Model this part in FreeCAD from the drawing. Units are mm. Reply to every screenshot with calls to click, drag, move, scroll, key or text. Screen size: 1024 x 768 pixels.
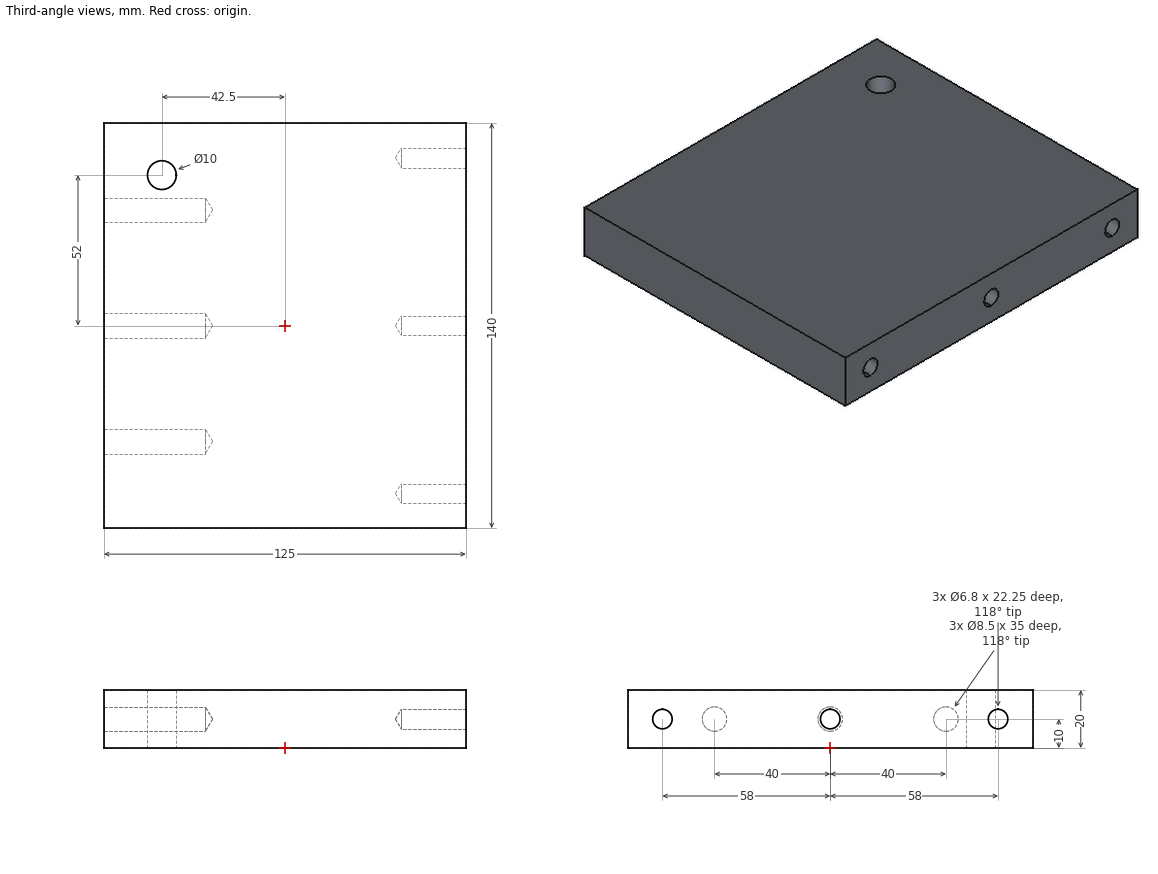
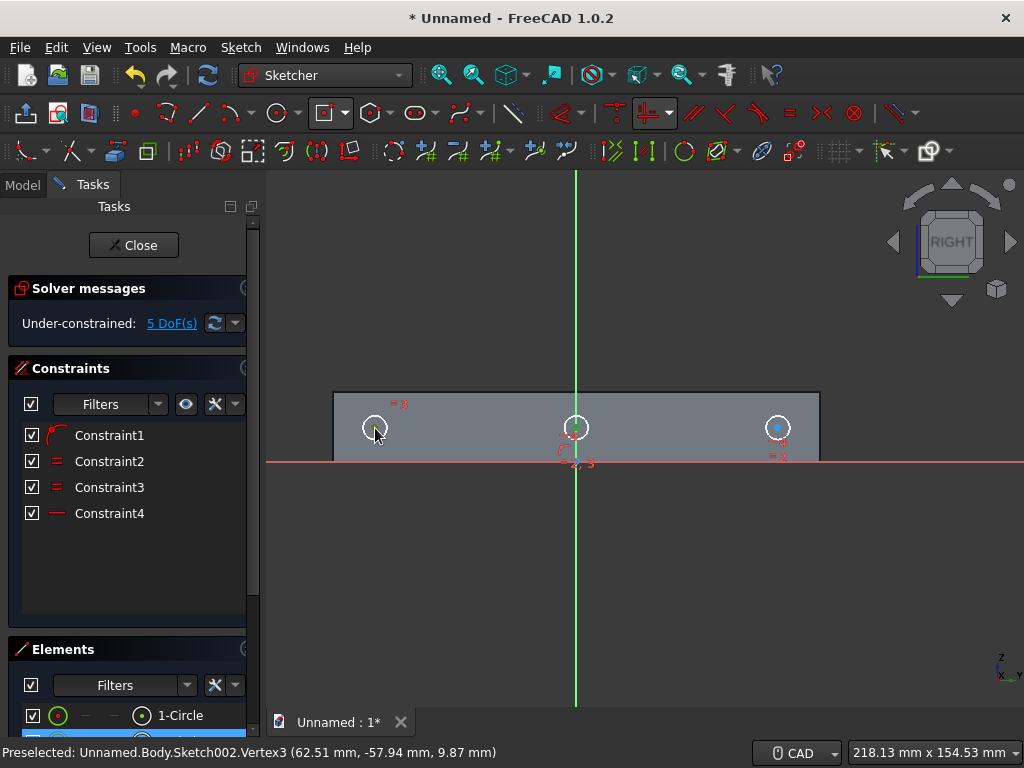
key(h)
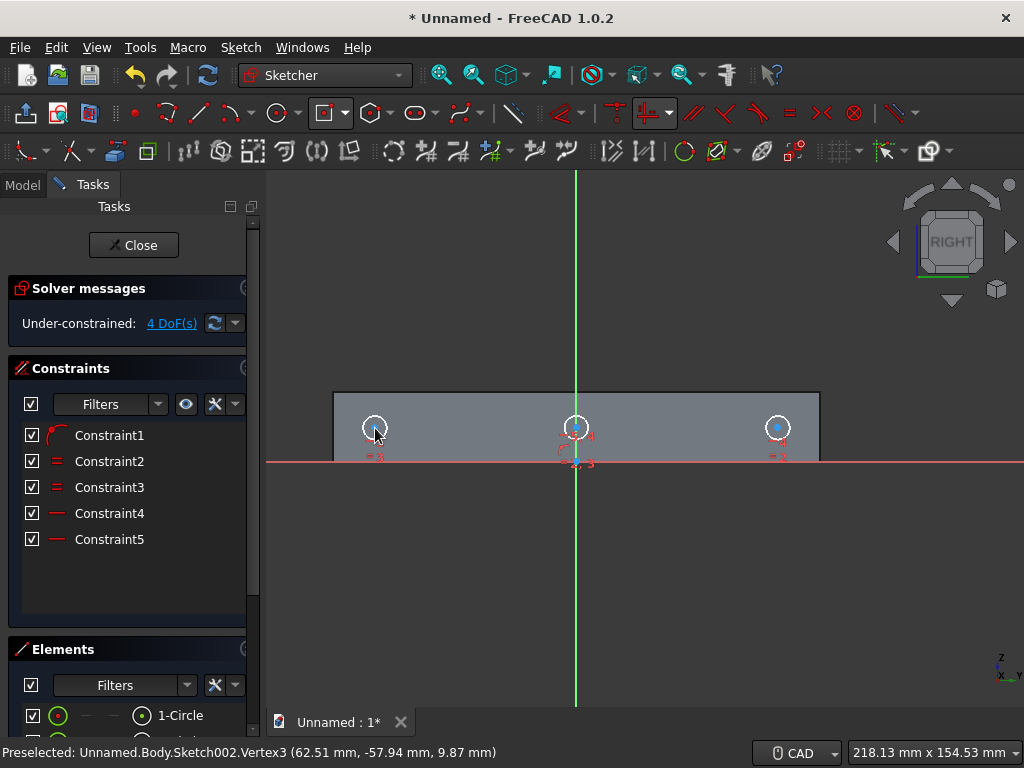
click(560, 114)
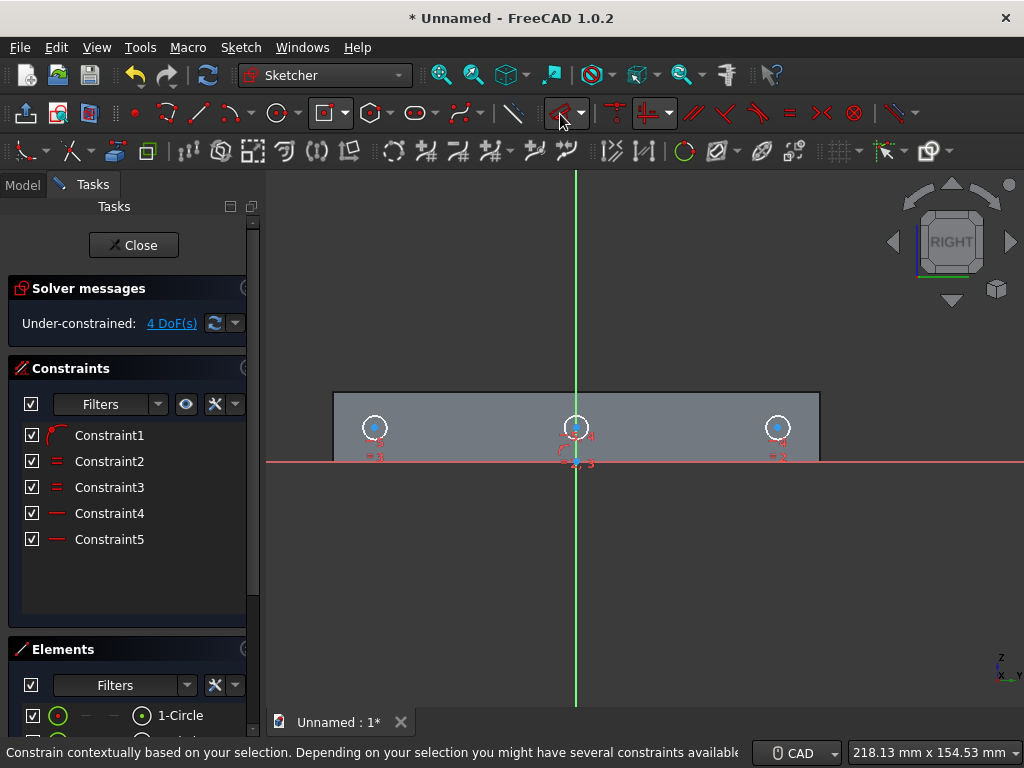
scroll(786, 419, up, 3)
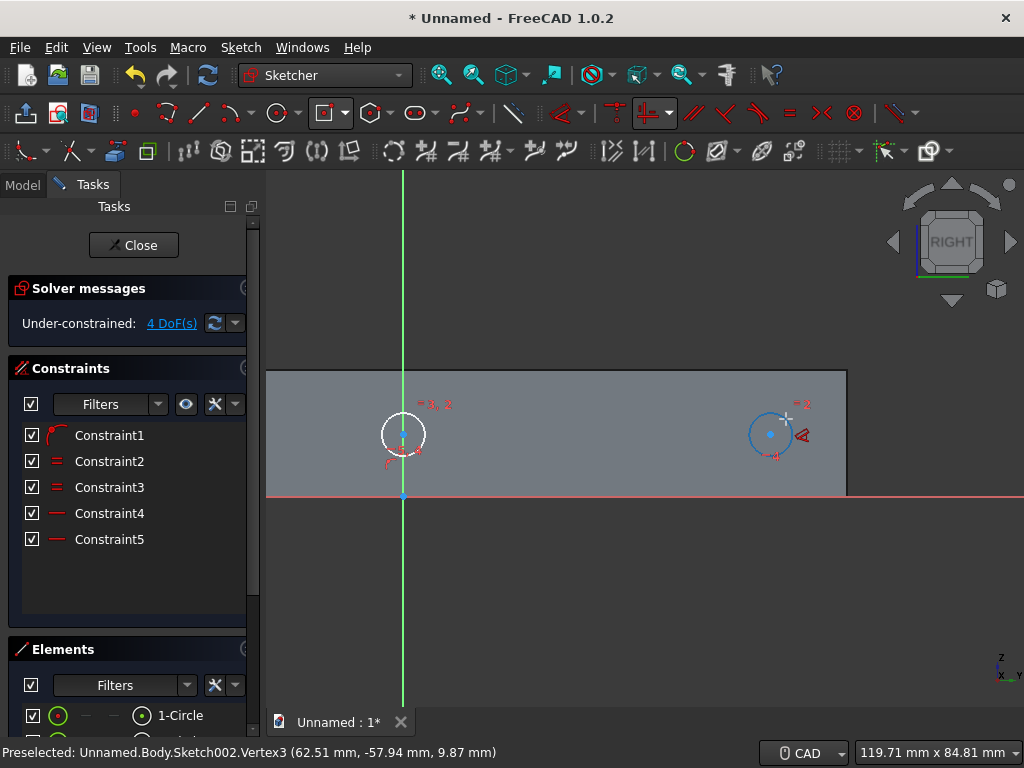
click(786, 419)
click(808, 396)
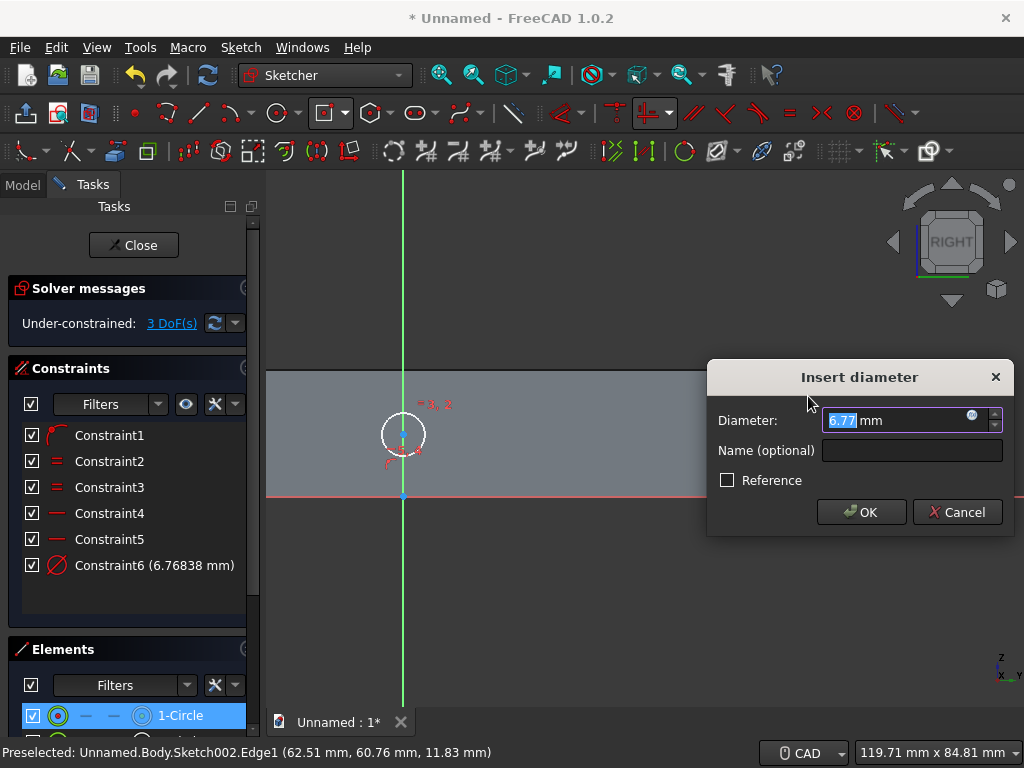
text(6.8)
key(Return)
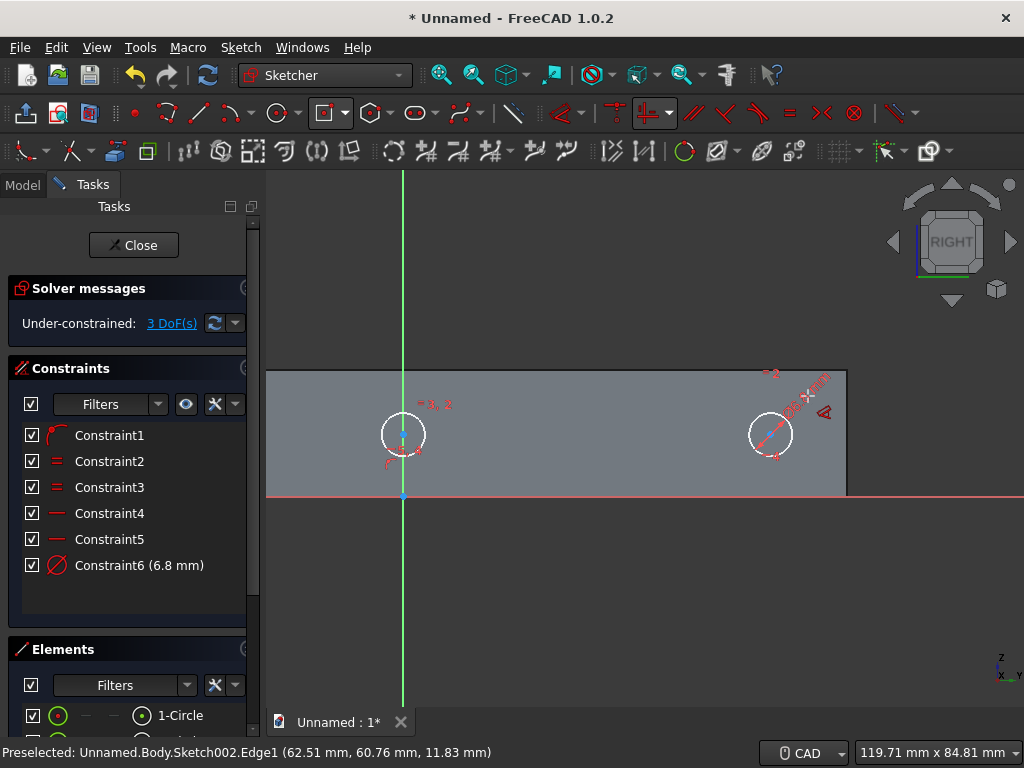
click(771, 435)
click(587, 531)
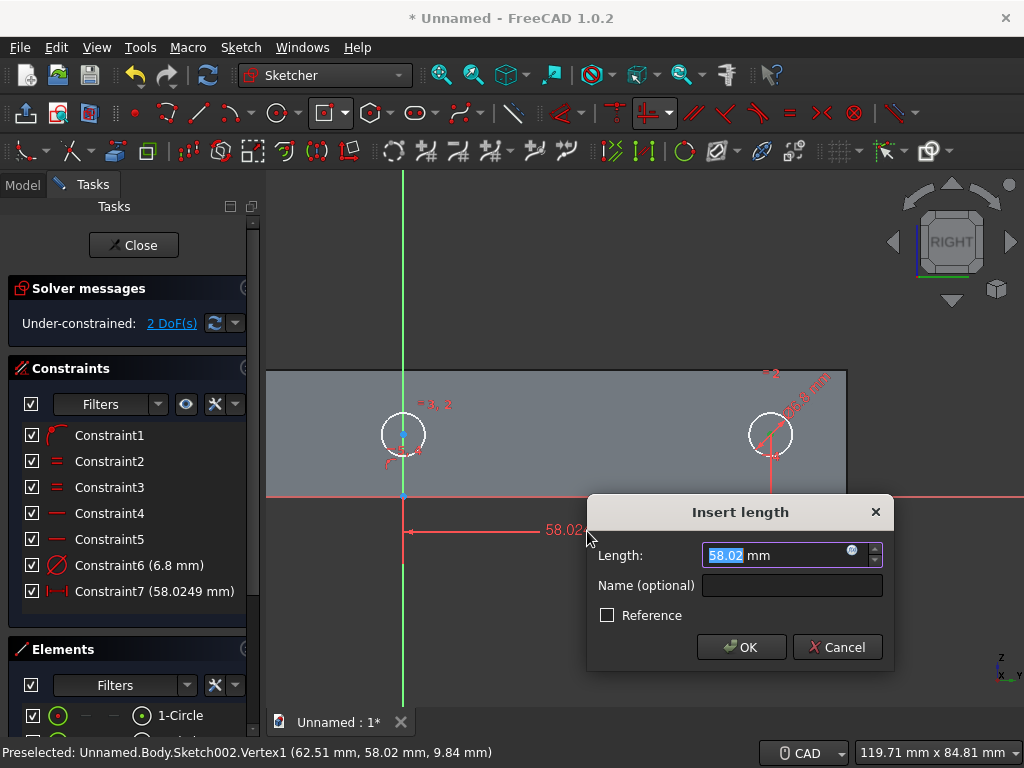
text(58)
key(Return)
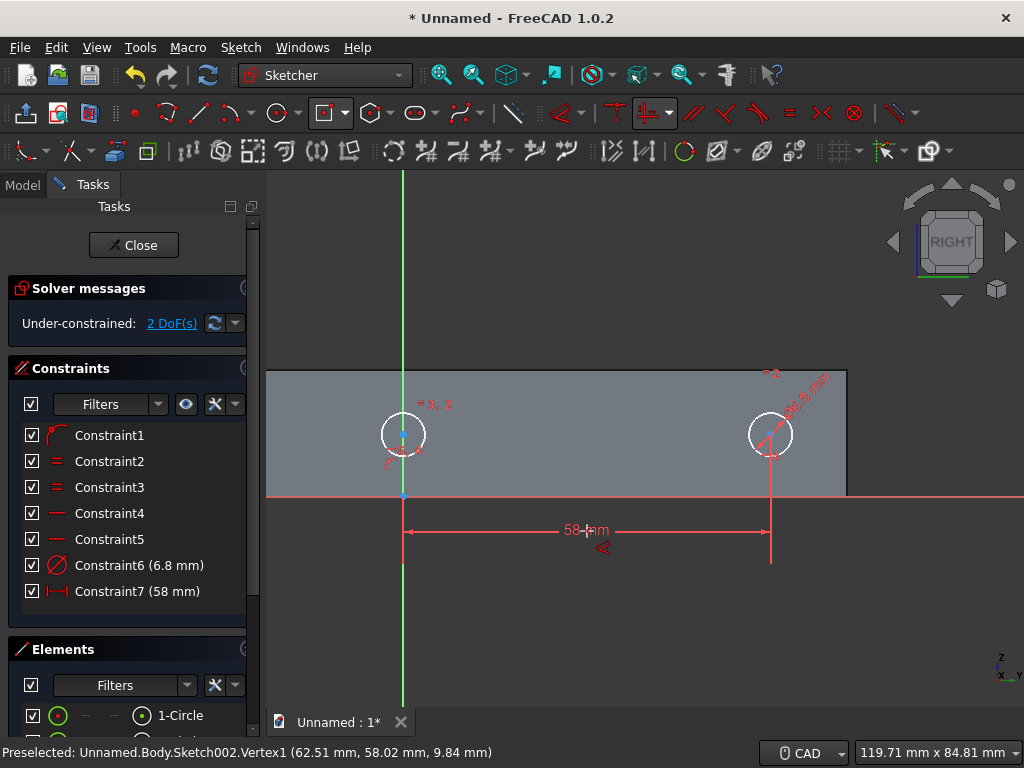
click(771, 435)
click(805, 466)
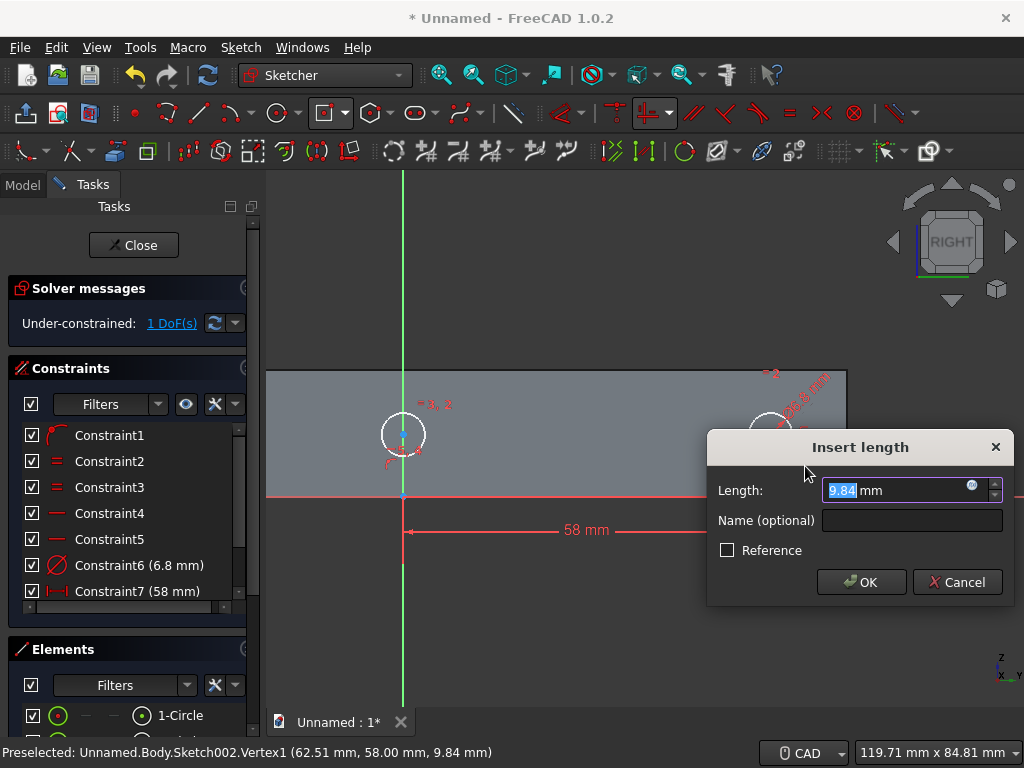
text(10)
key(Return)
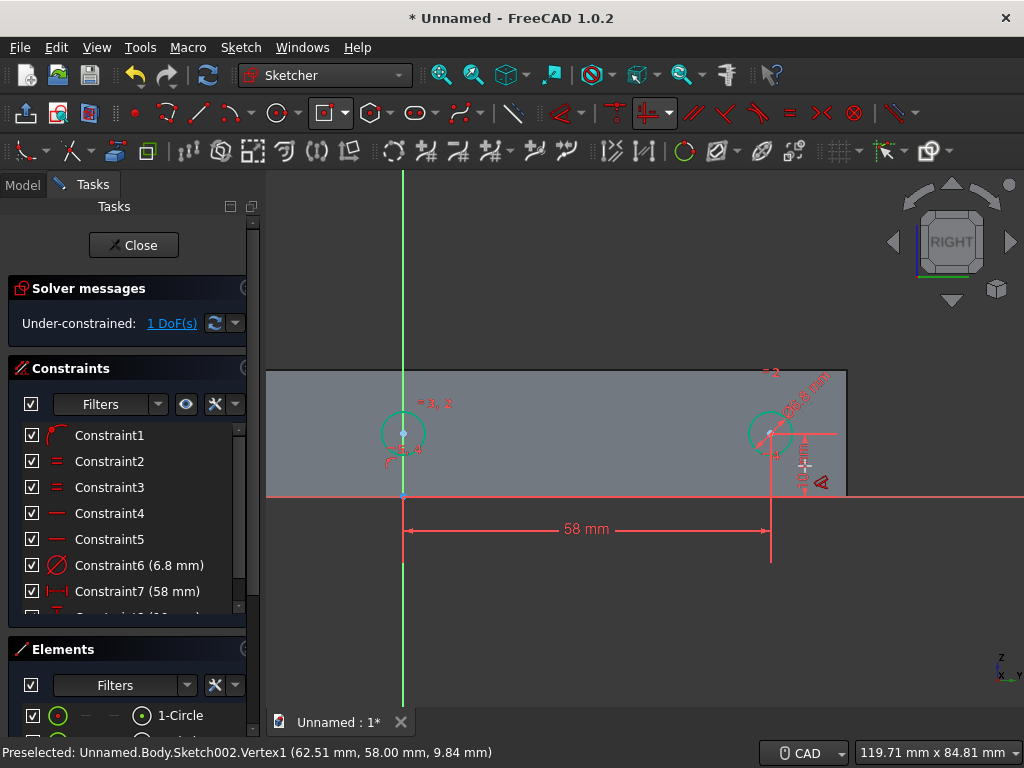
scroll(787, 419, down, 3)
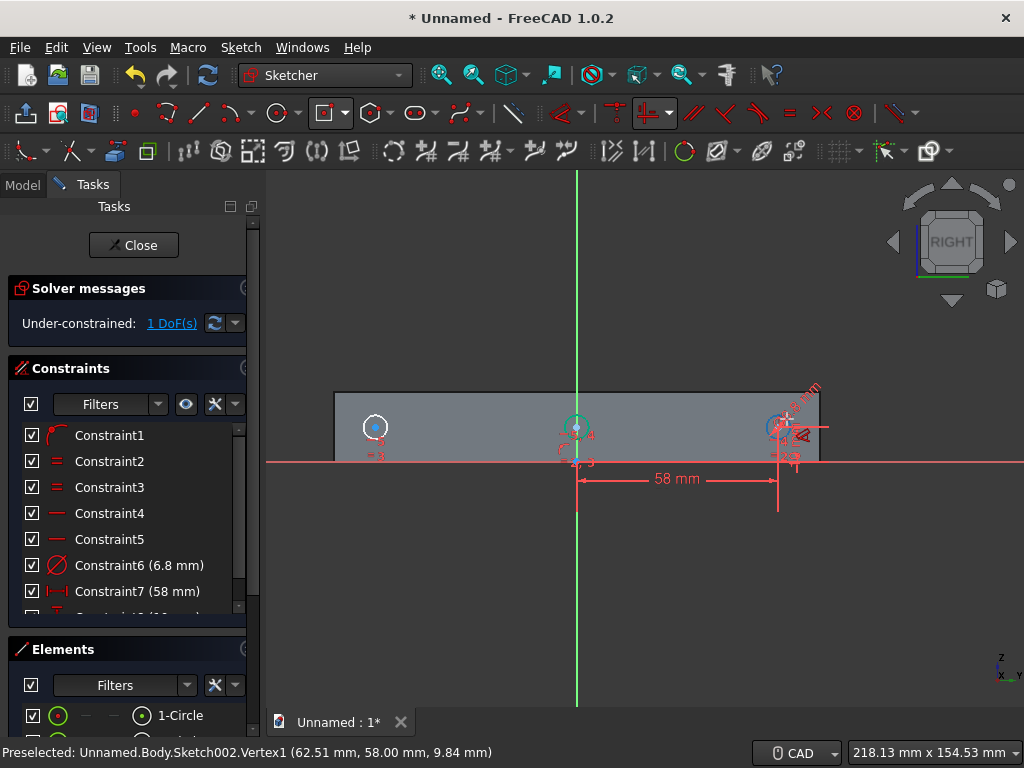
click(375, 427)
click(476, 496)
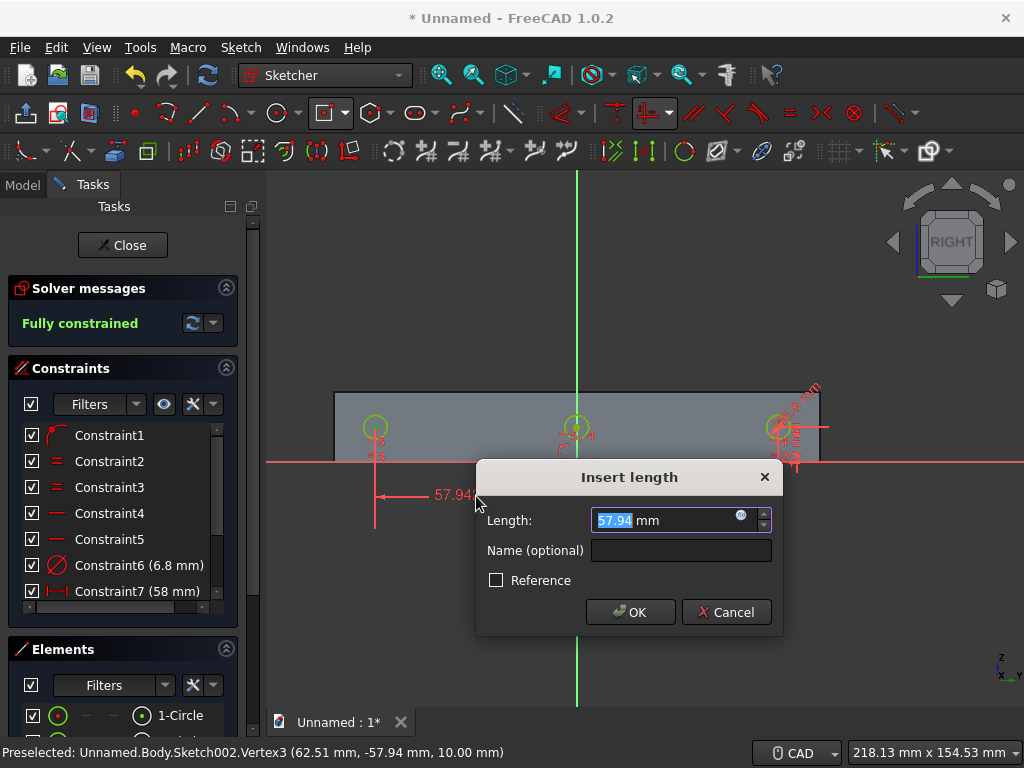
text(58)
key(Return)
key(Escape)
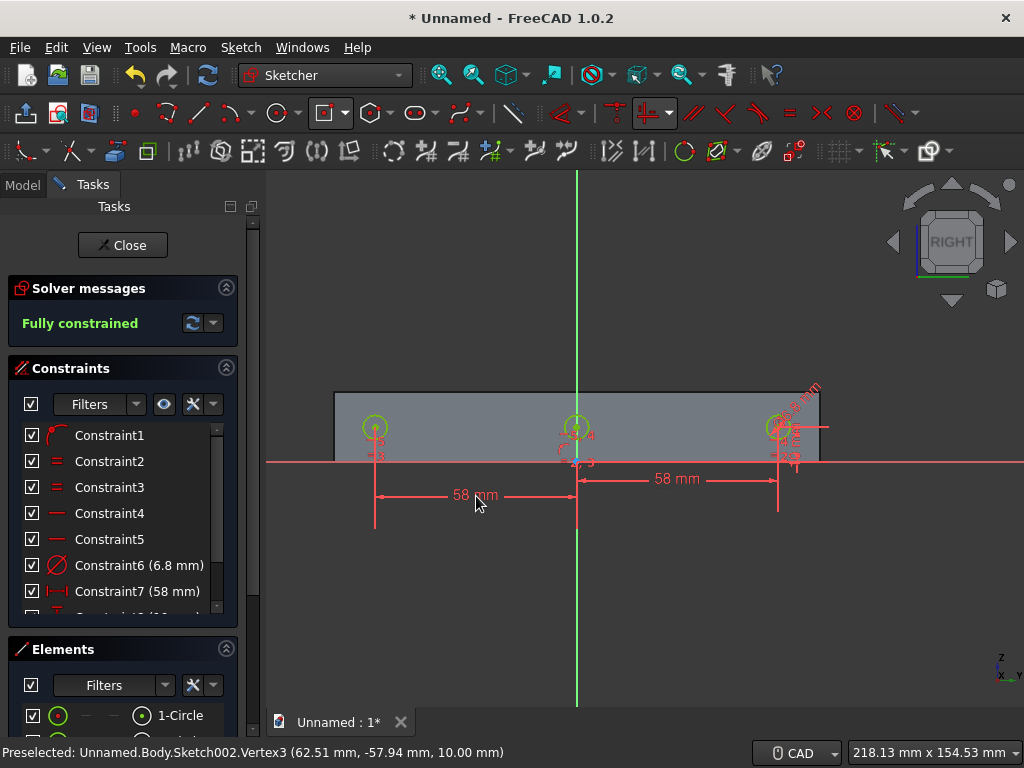
click(123, 245)